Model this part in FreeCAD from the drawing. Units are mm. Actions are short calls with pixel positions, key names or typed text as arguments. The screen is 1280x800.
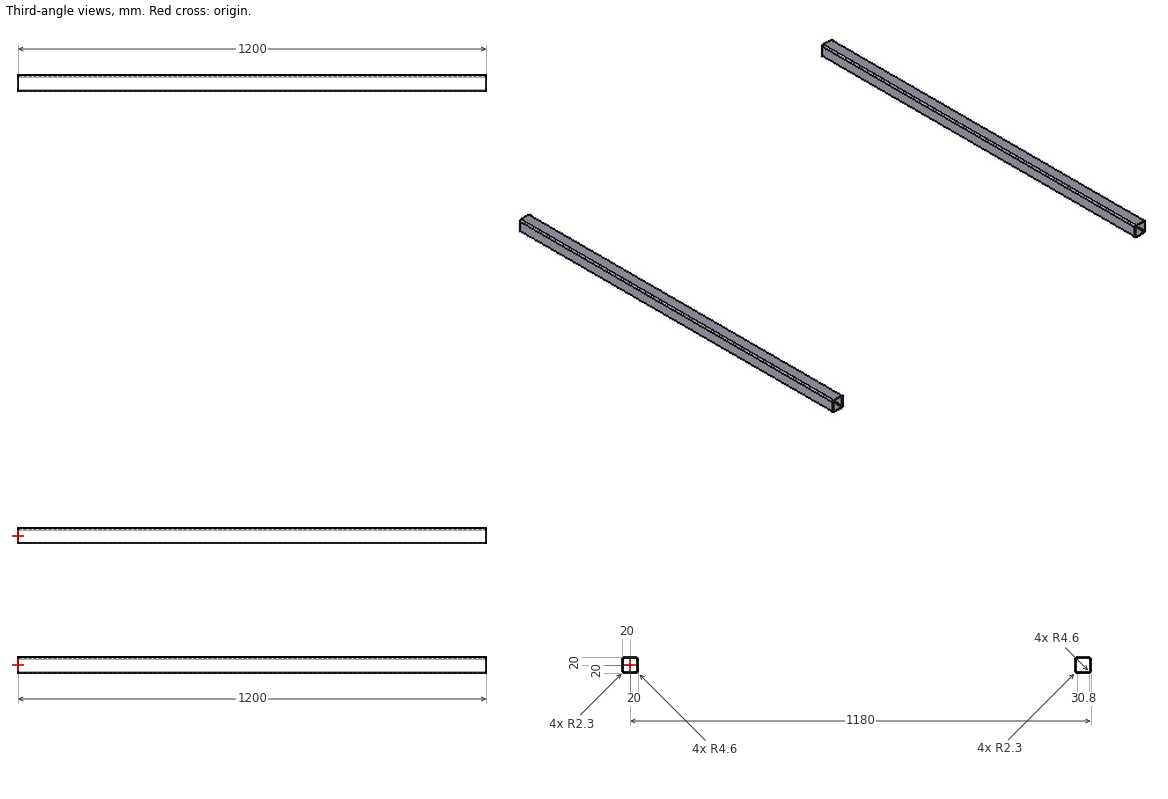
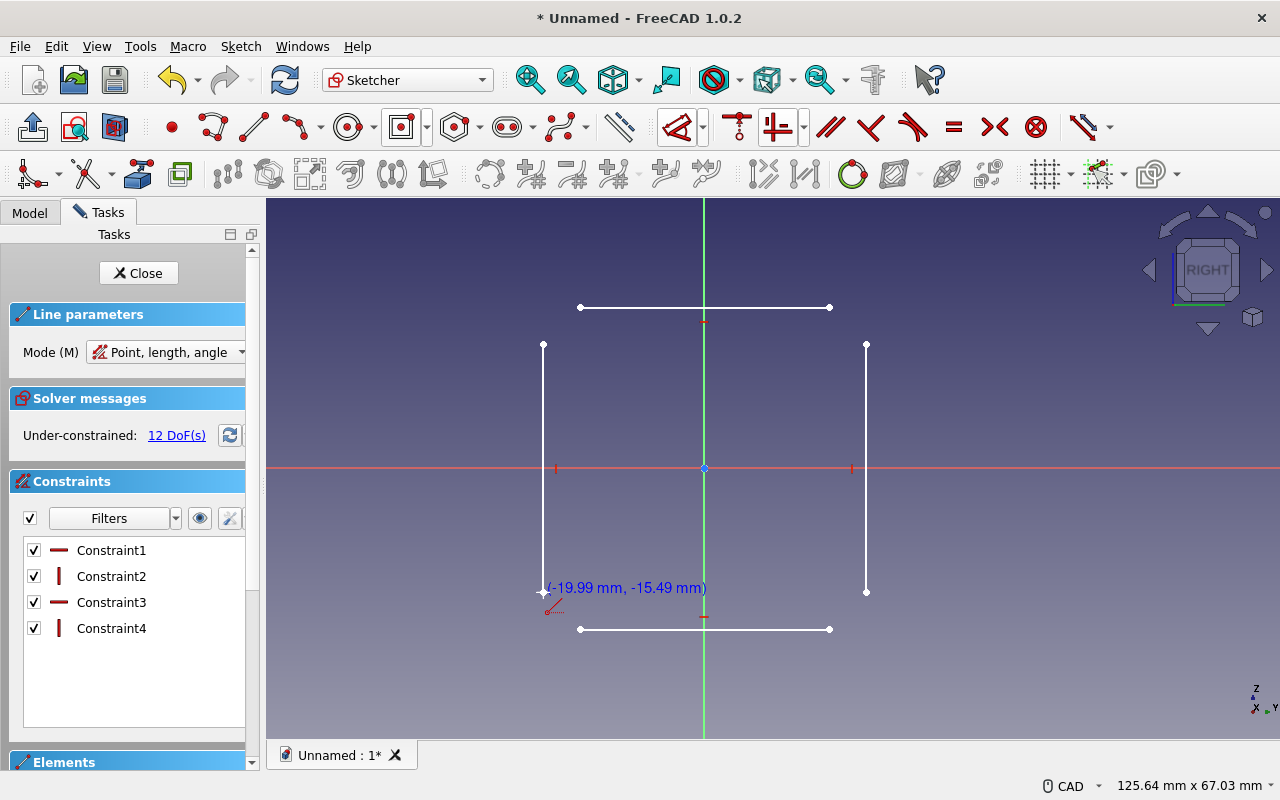
click(294, 128)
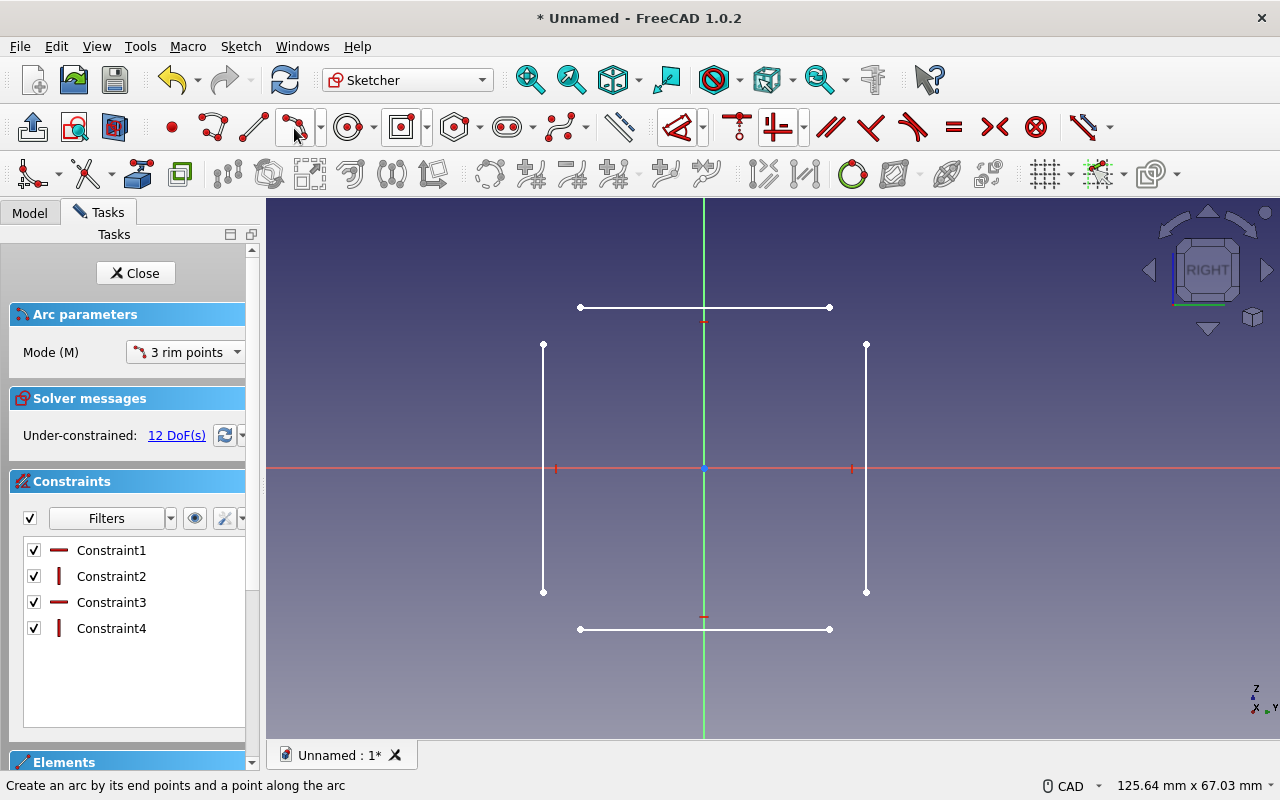
click(829, 630)
click(866, 593)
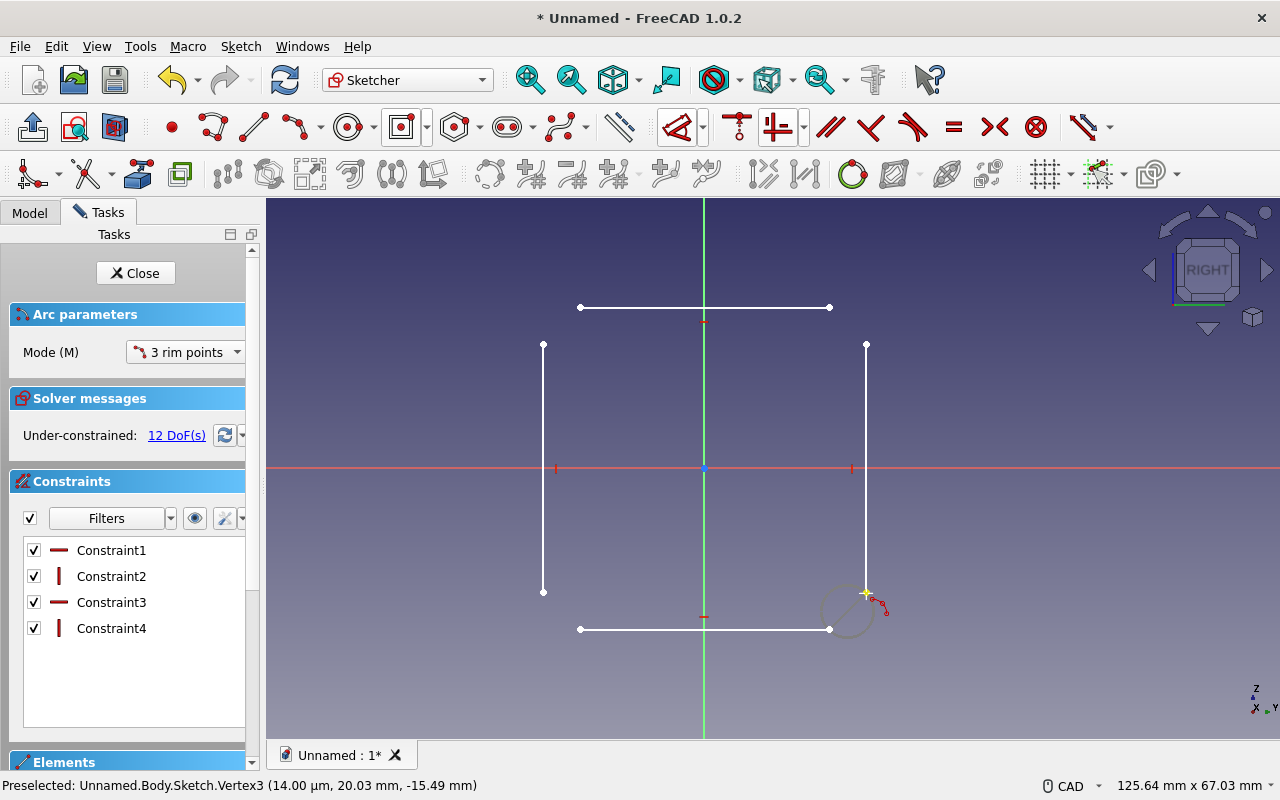
scroll(855, 619, up, 2)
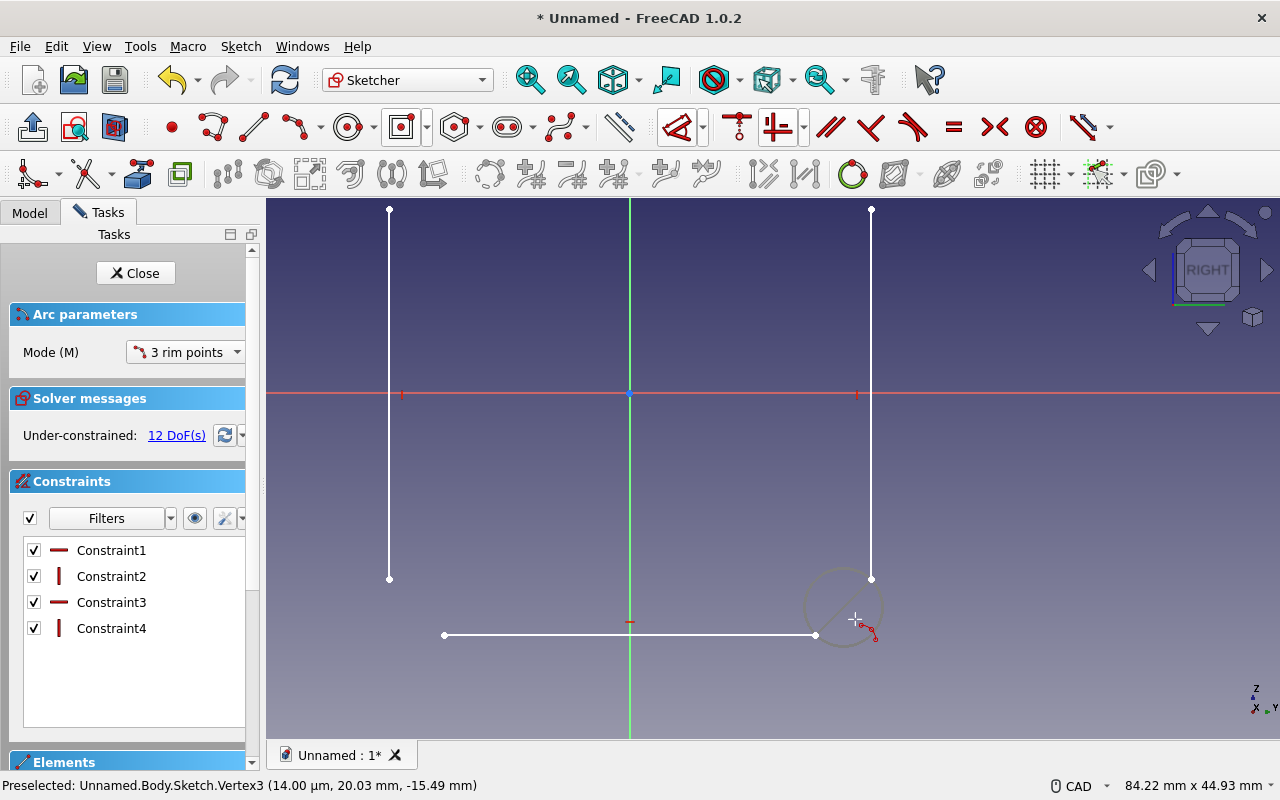
click(855, 618)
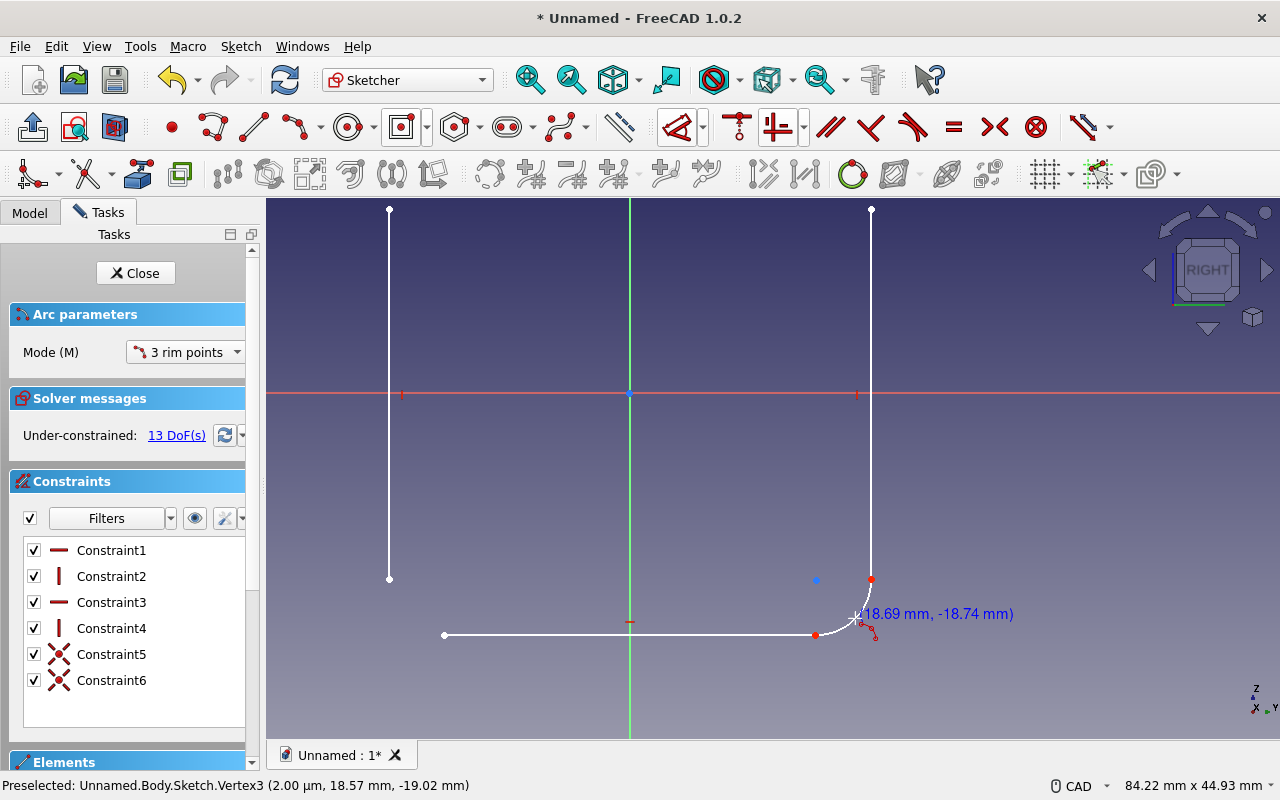
scroll(856, 621, down, 2)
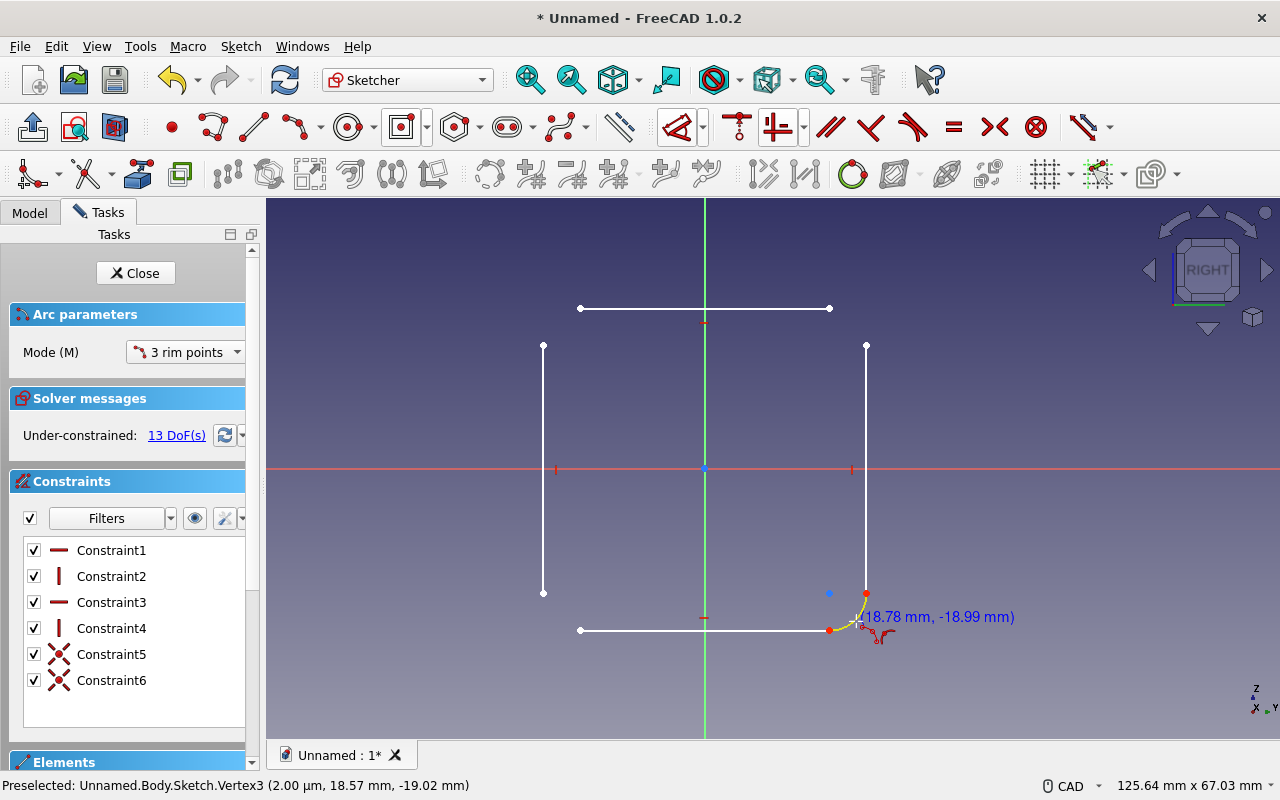
click(866, 346)
click(829, 309)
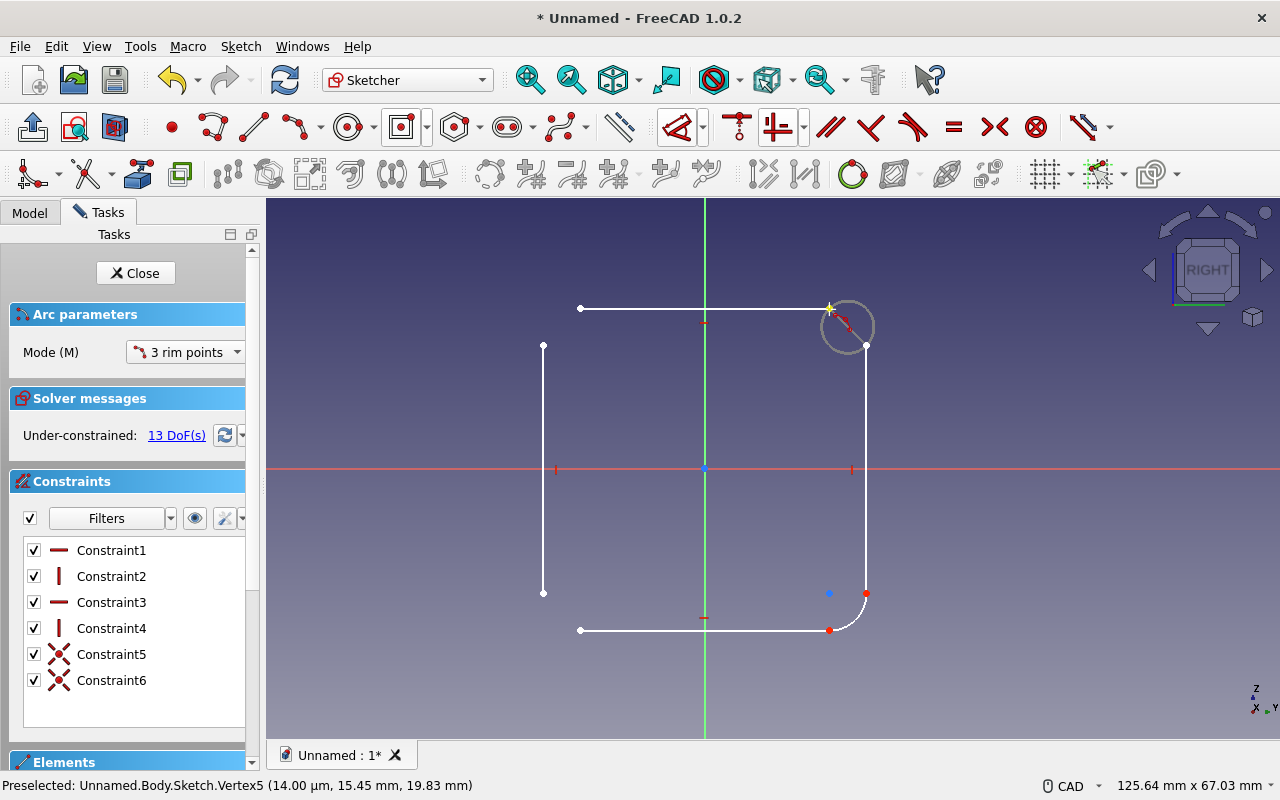
scroll(855, 318, up, 2)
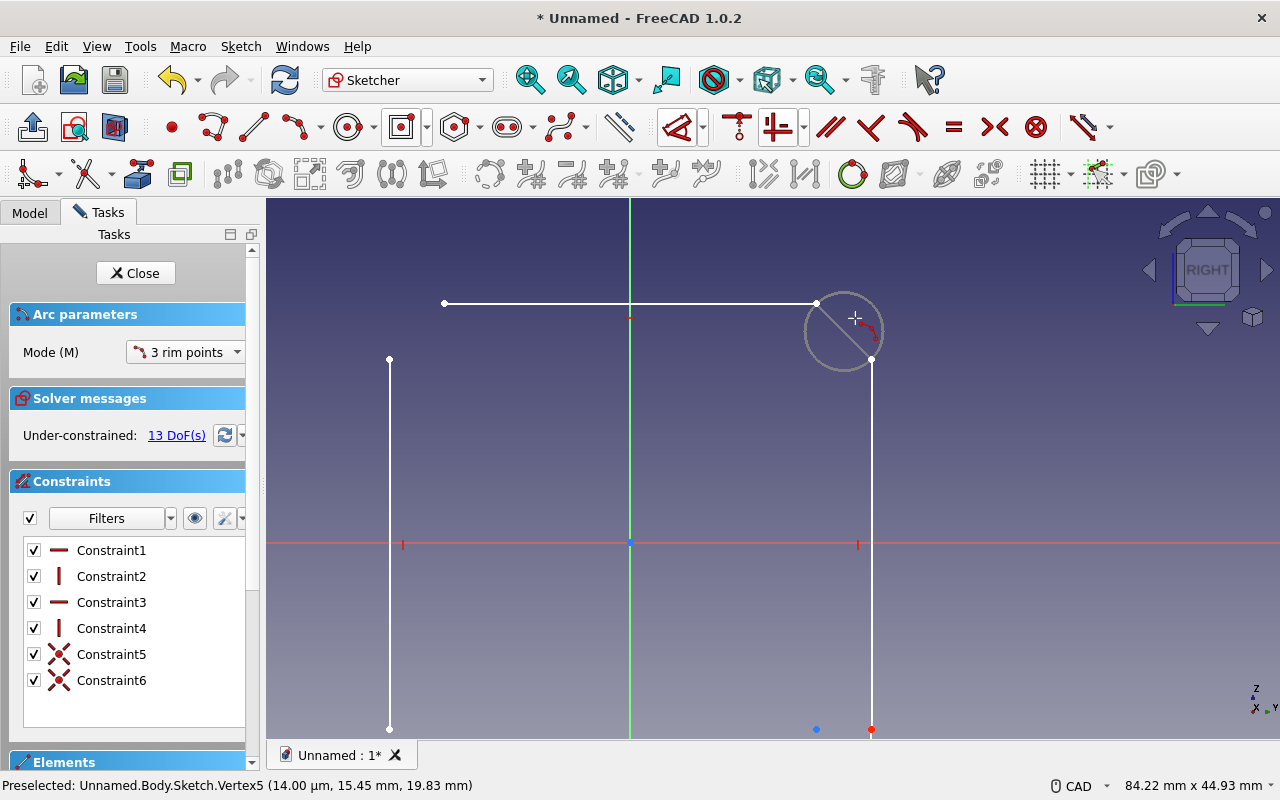
click(855, 318)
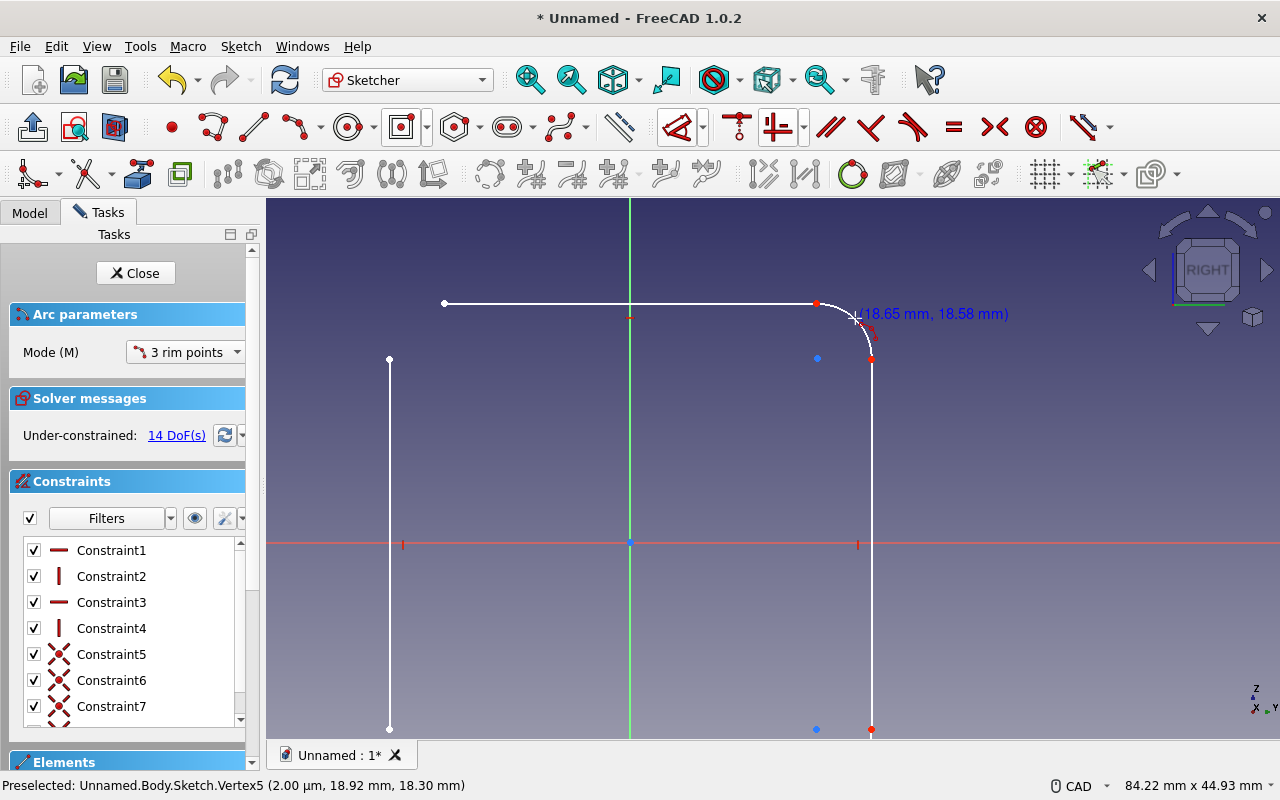
click(445, 304)
click(390, 359)
click(406, 318)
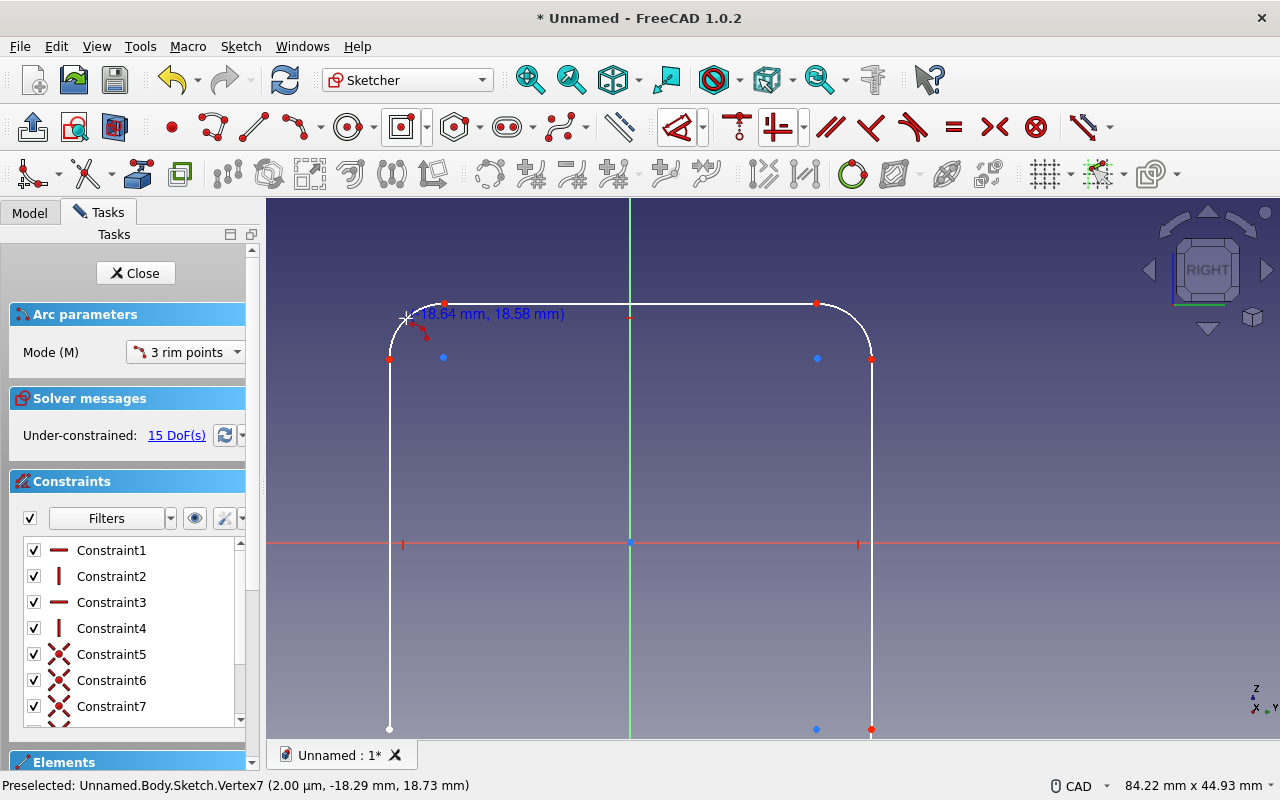
scroll(855, 318, down, 2)